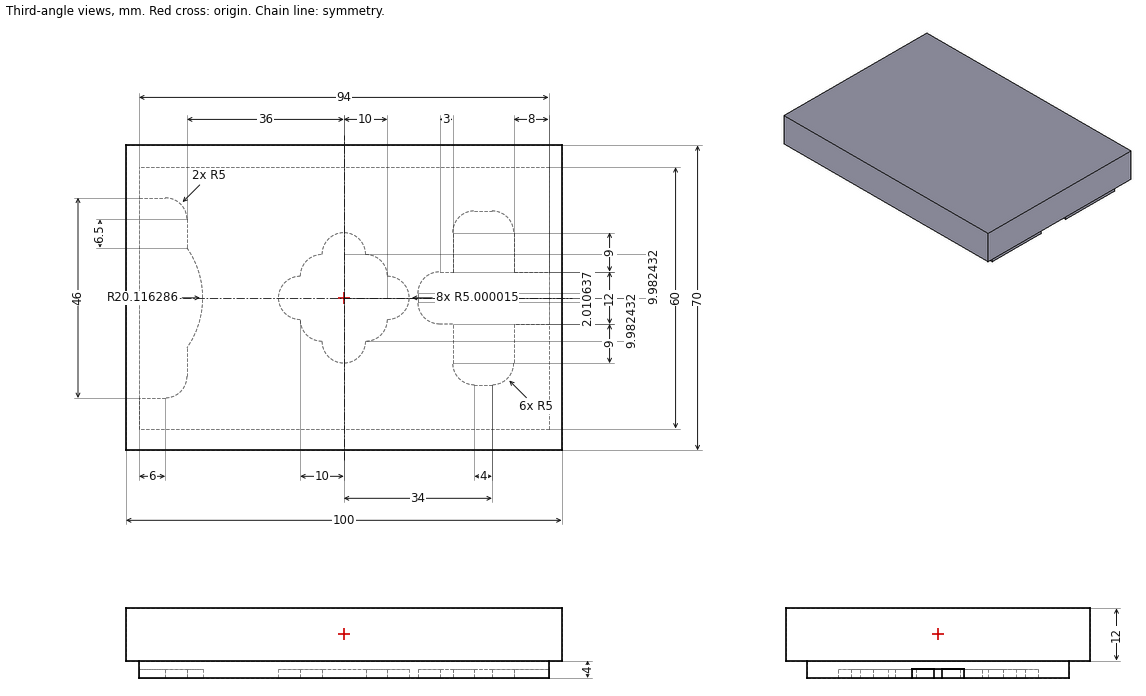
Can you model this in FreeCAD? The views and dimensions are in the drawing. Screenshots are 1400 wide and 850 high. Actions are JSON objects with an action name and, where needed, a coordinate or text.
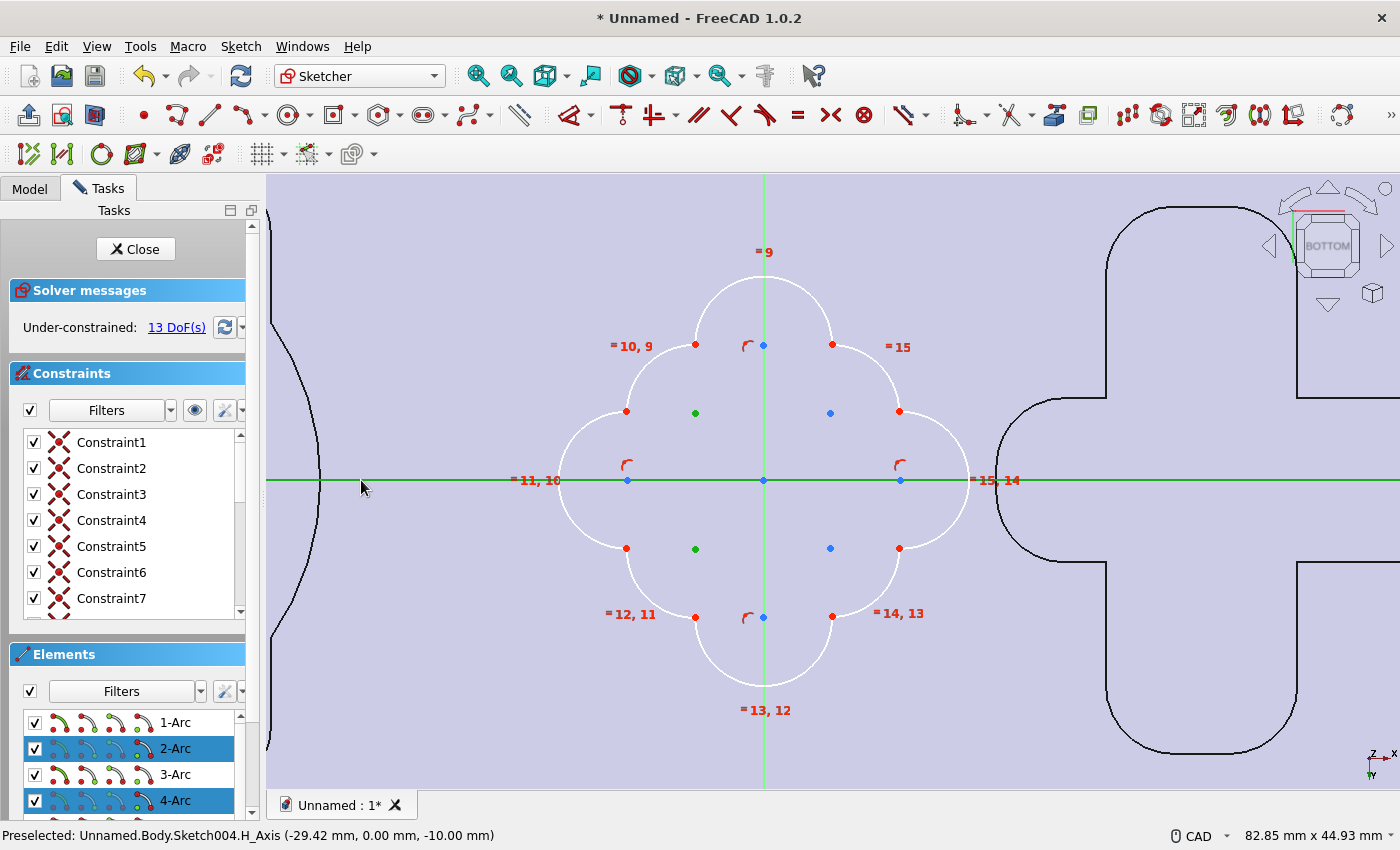
{"action": "left_click", "coordinate": [831, 116]}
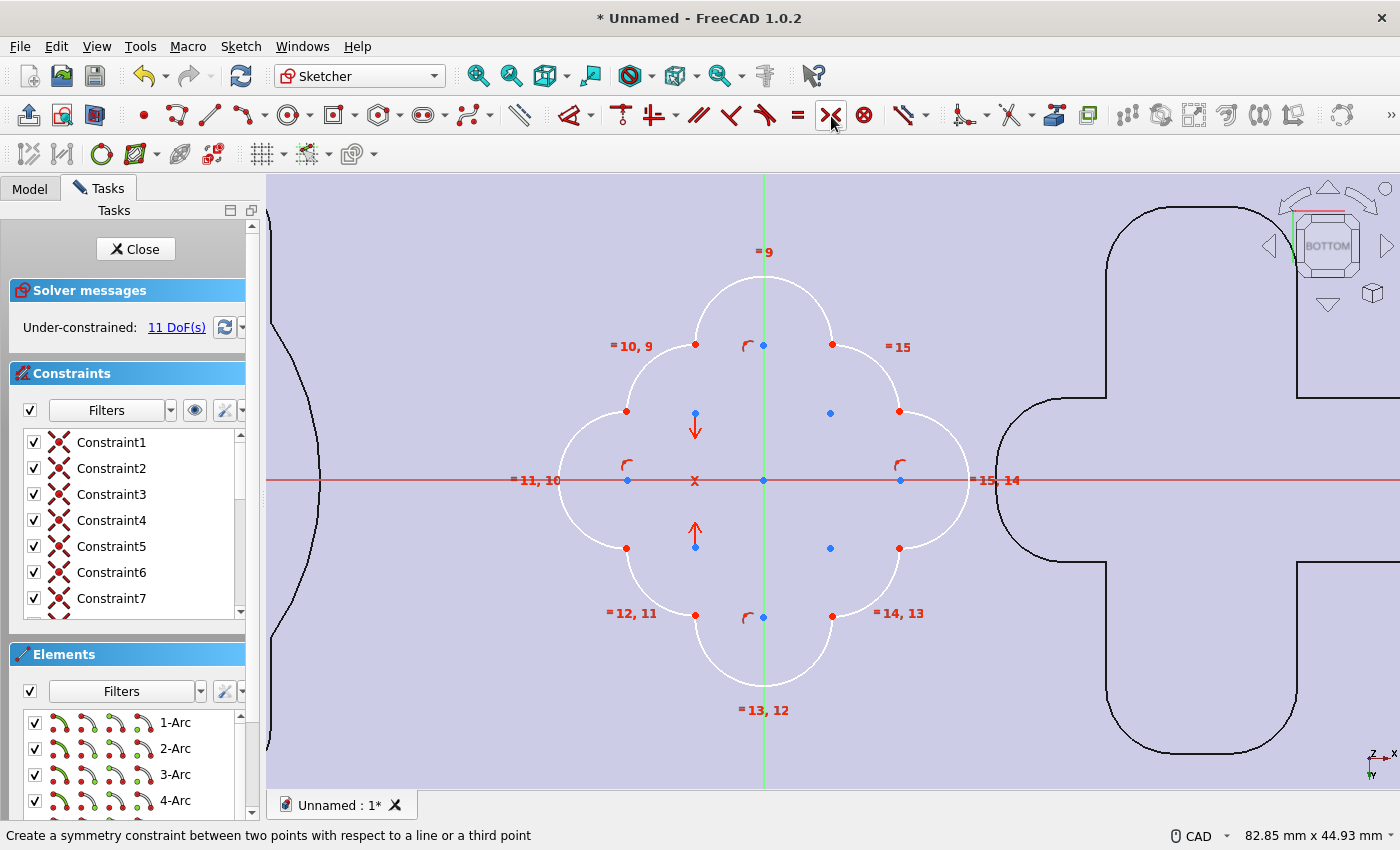
{"action": "left_click", "coordinate": [695, 547]}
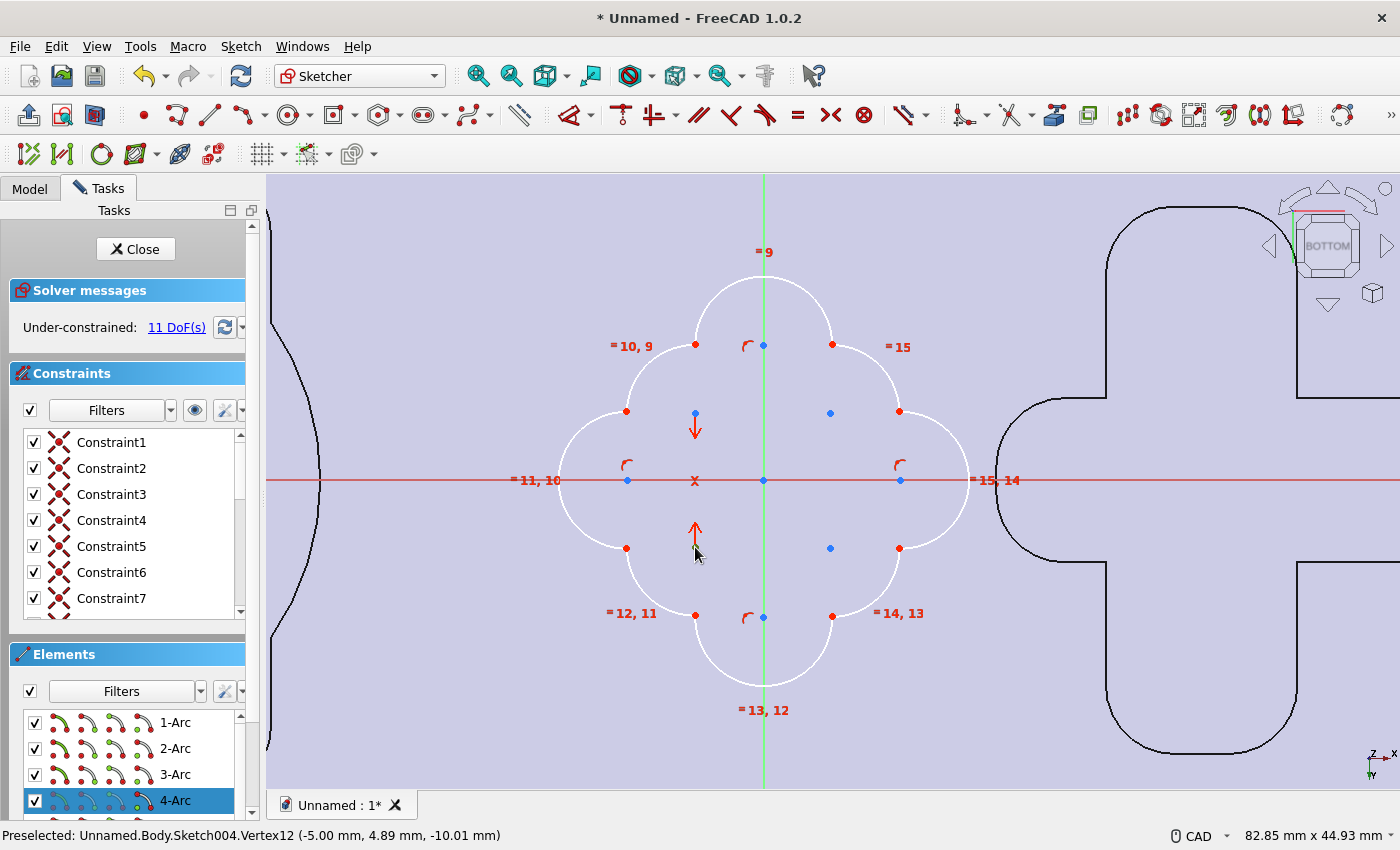
{"action": "left_click", "coordinate": [831, 549]}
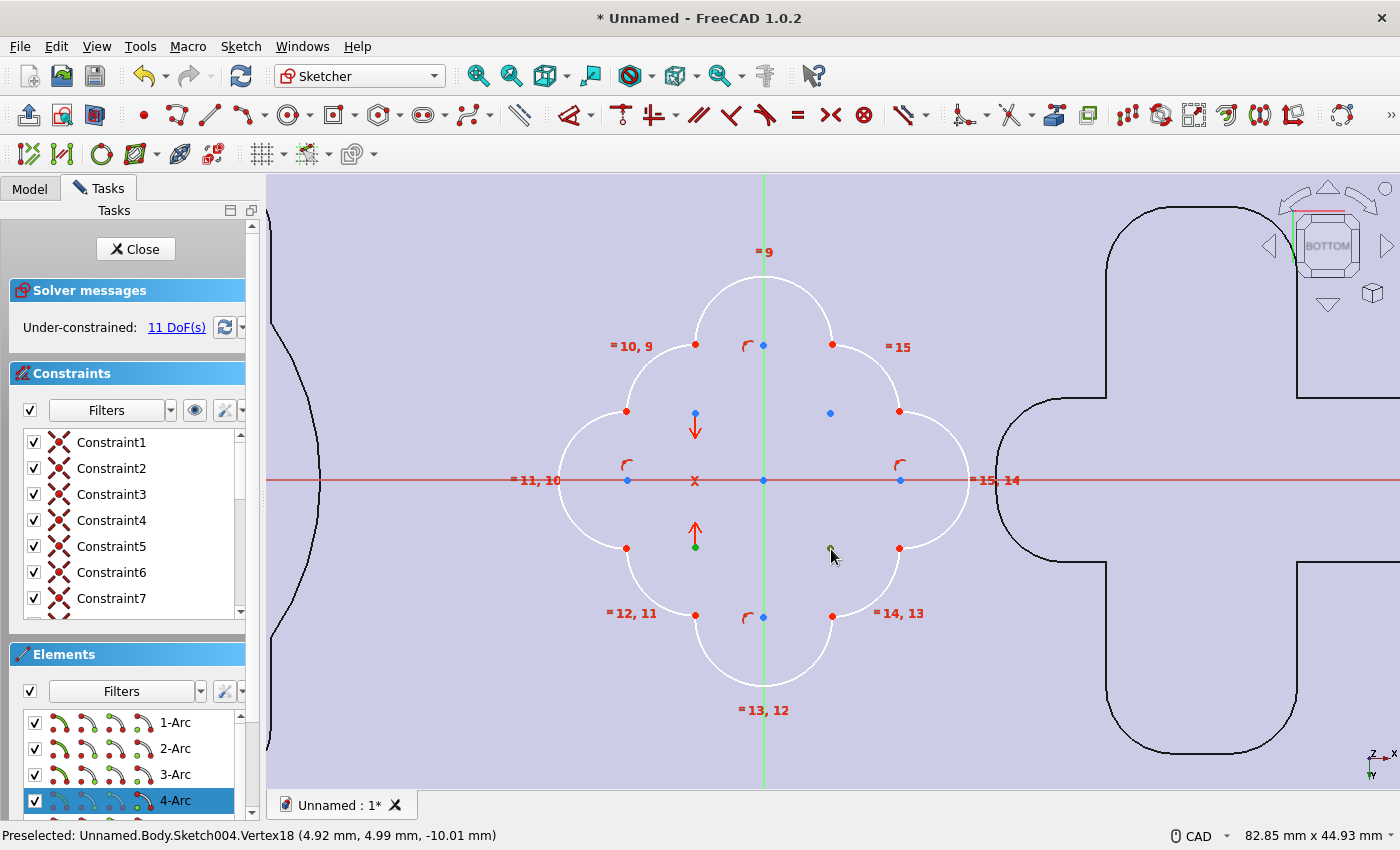
{"action": "left_click", "coordinate": [764, 721]}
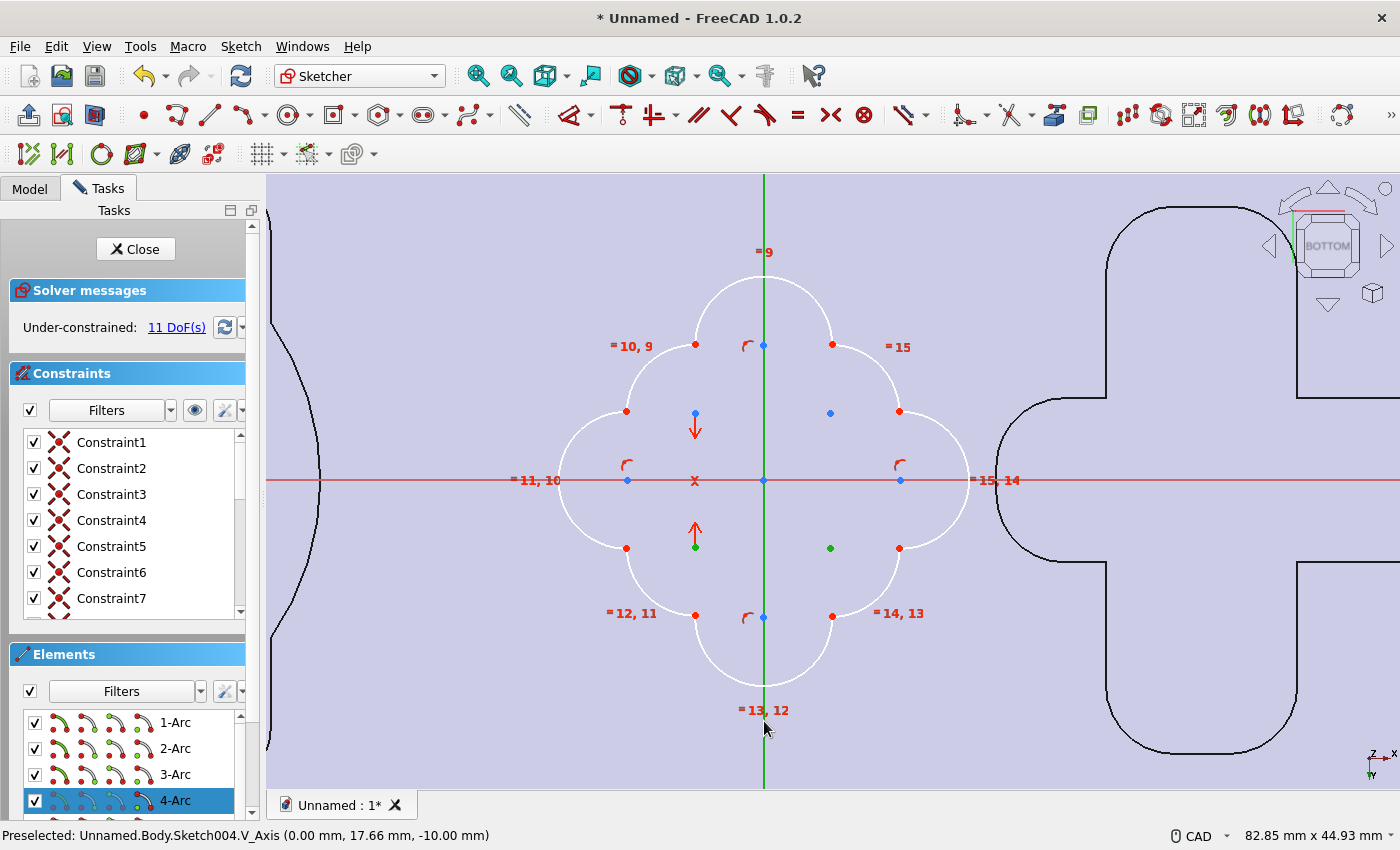
{"action": "left_click", "coordinate": [831, 116]}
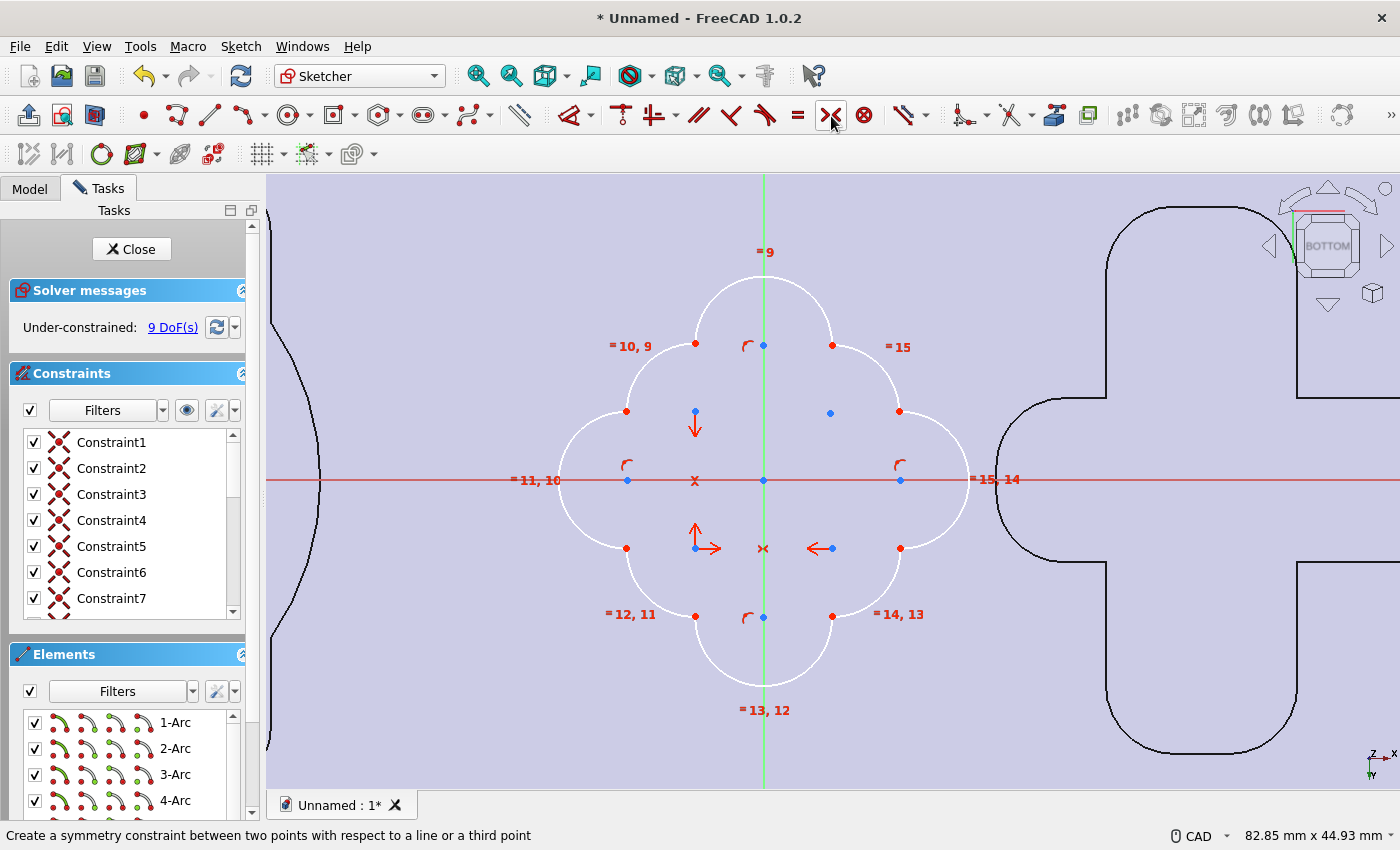
{"action": "left_click", "coordinate": [695, 412]}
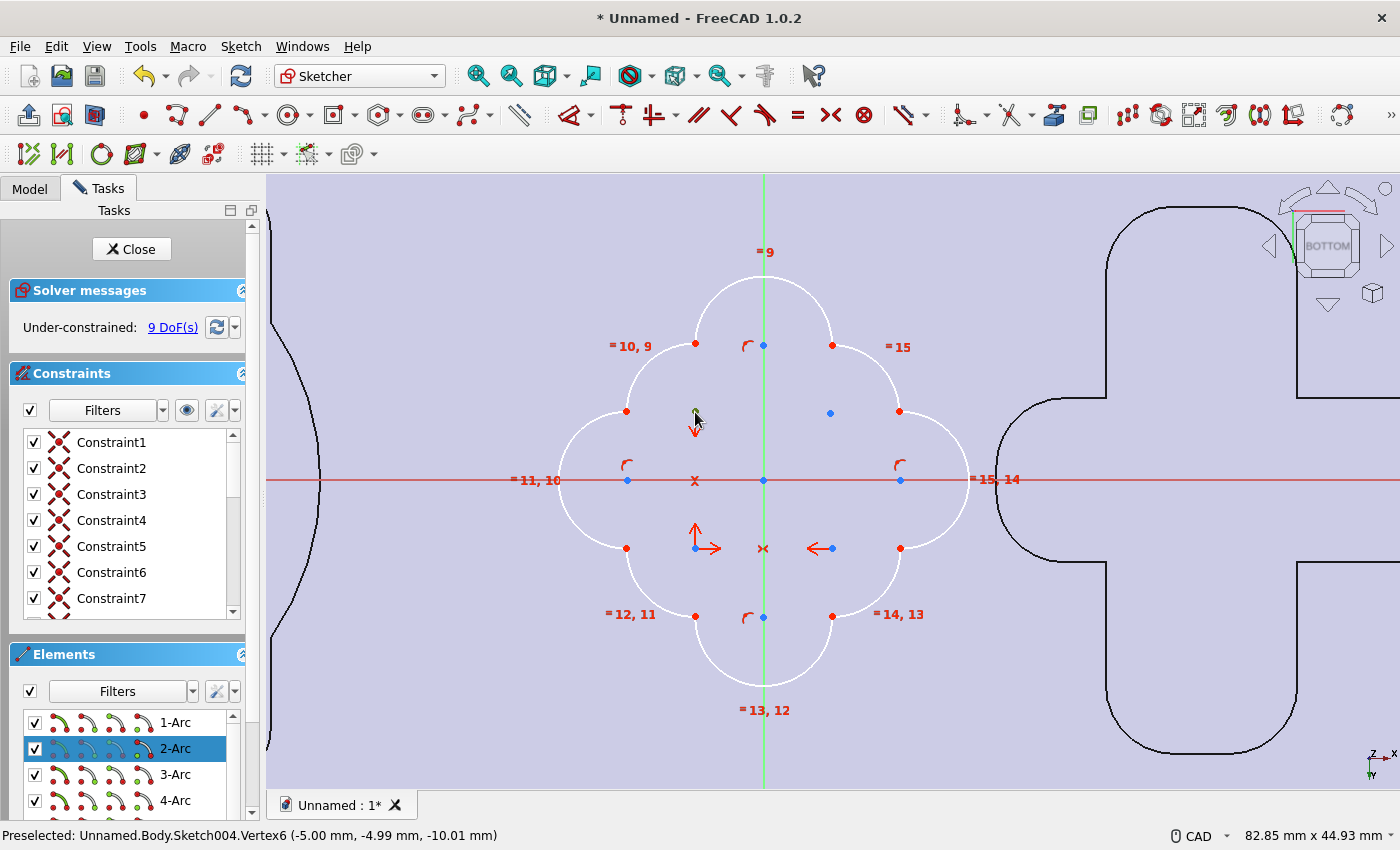
{"action": "left_click", "coordinate": [831, 413]}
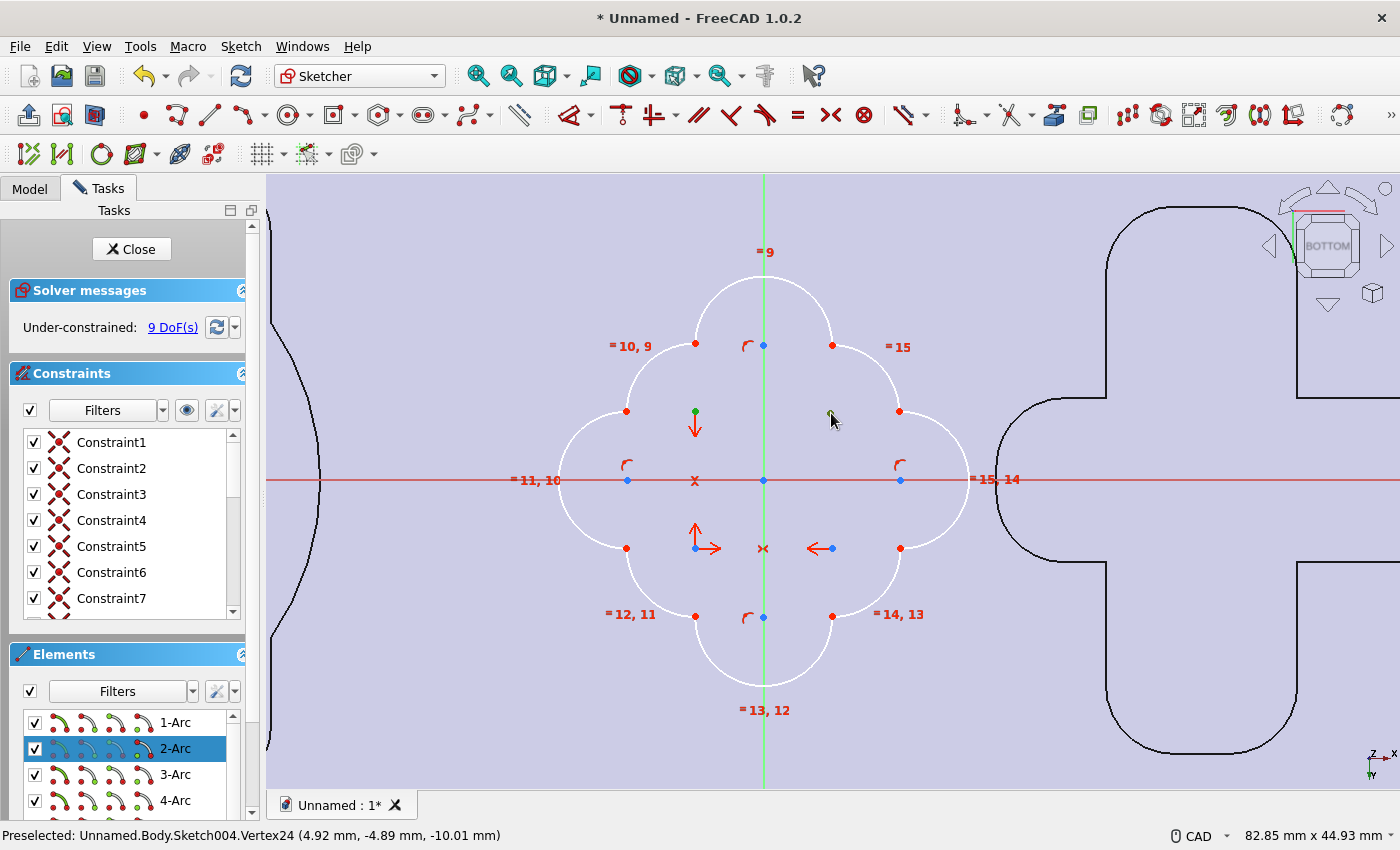
{"action": "left_click", "coordinate": [764, 721]}